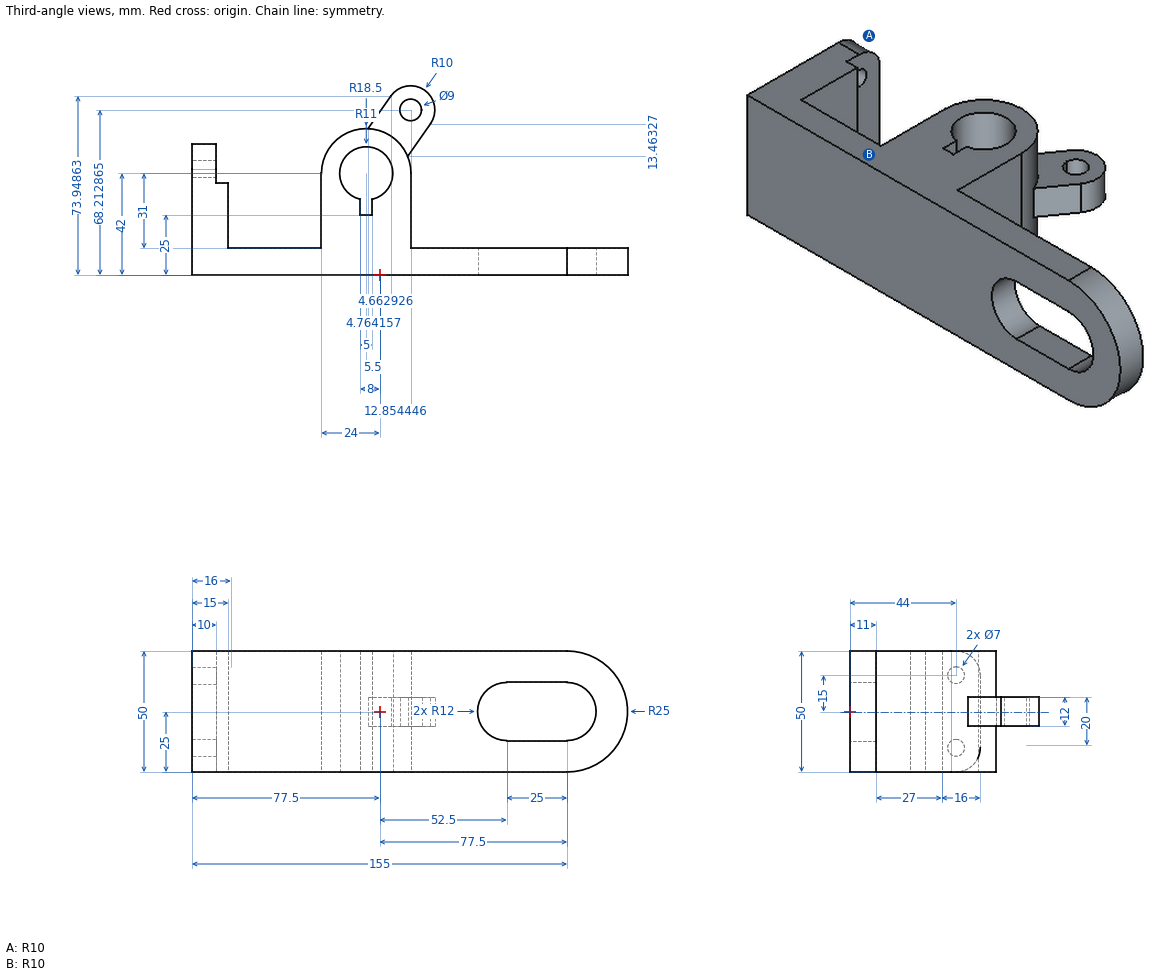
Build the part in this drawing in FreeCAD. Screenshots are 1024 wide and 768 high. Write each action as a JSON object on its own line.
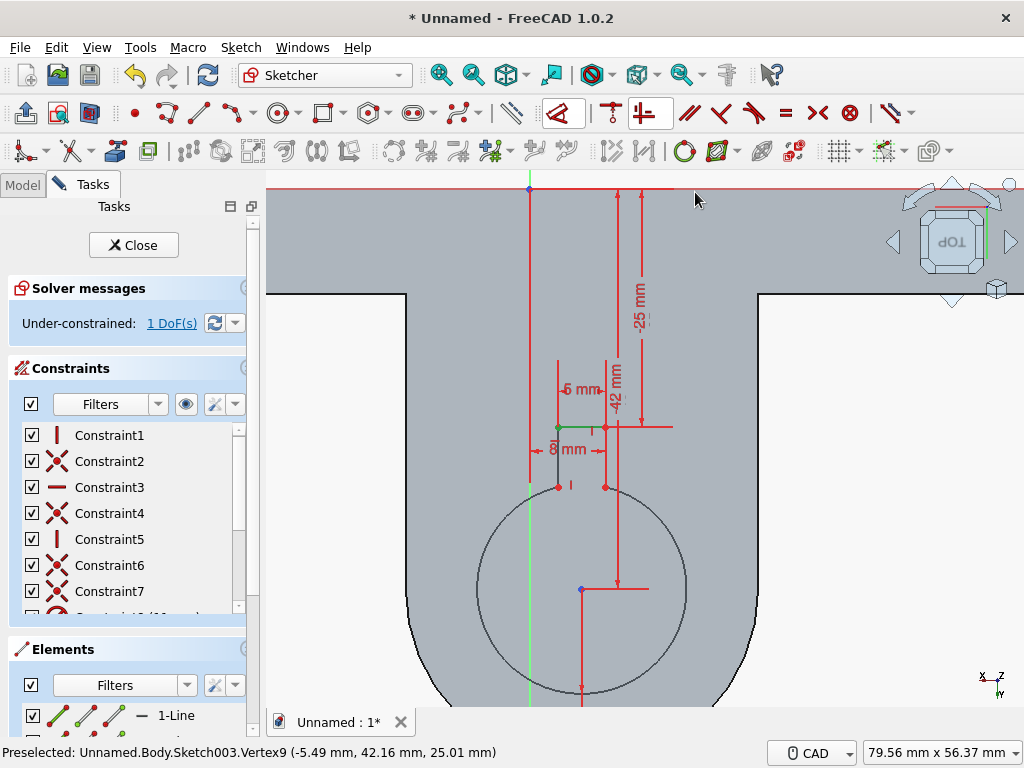
{"action": "left_click", "coordinate": [582, 589]}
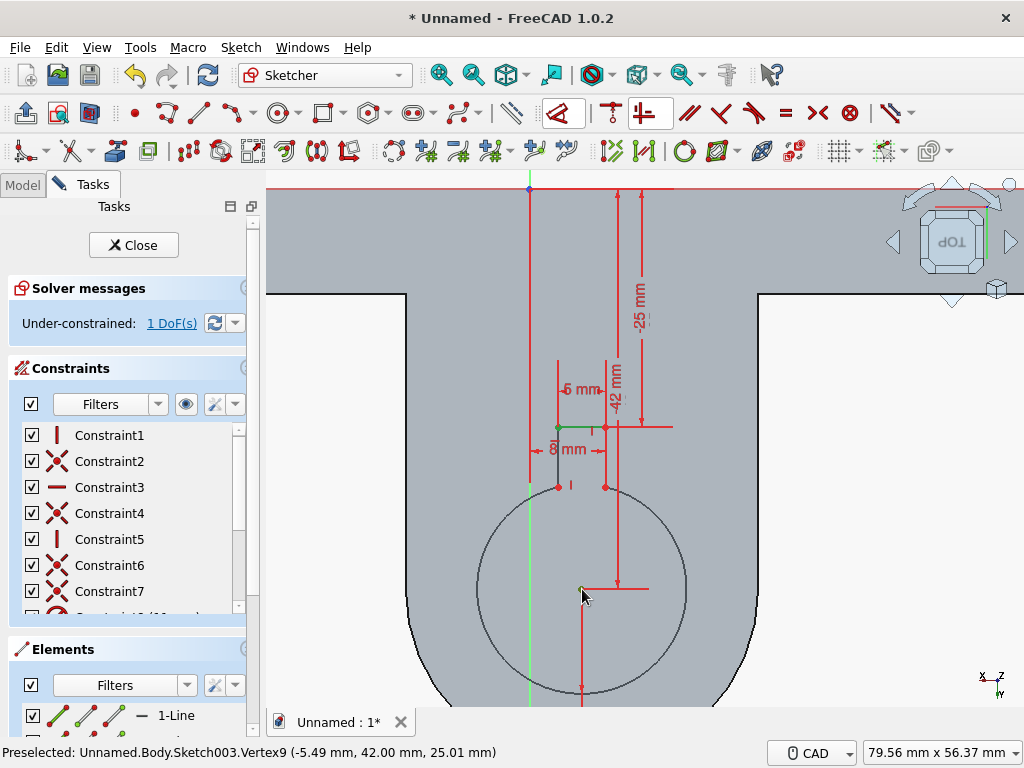
{"action": "left_click", "coordinate": [580, 114]}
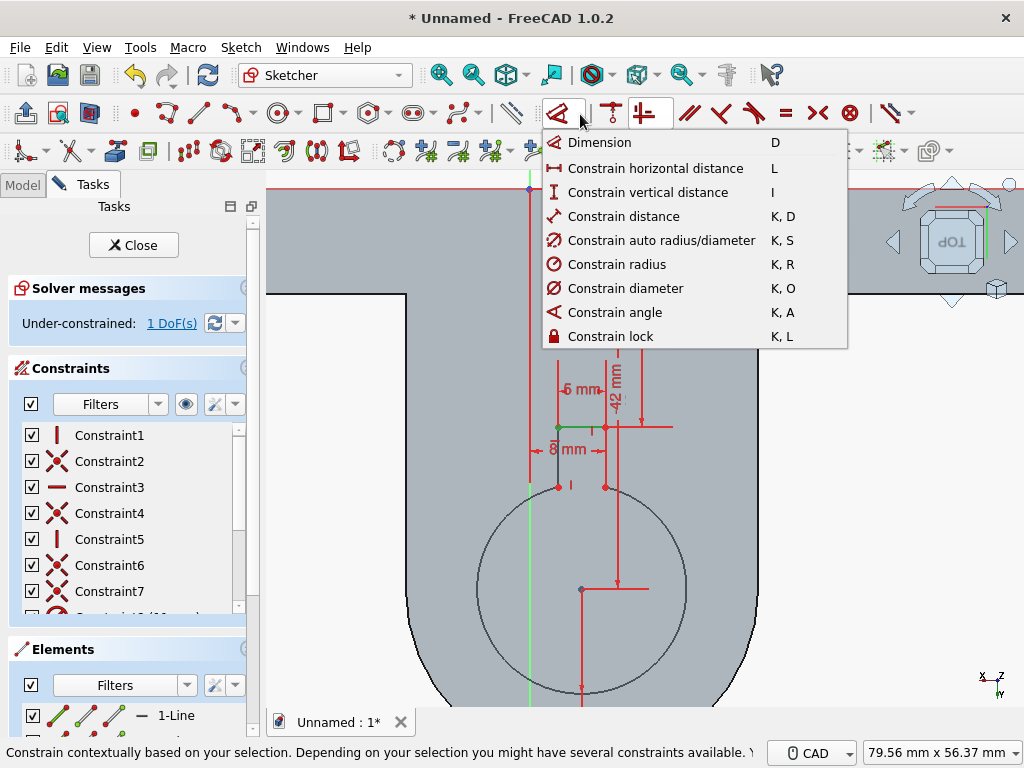
{"action": "left_click", "coordinate": [695, 168]}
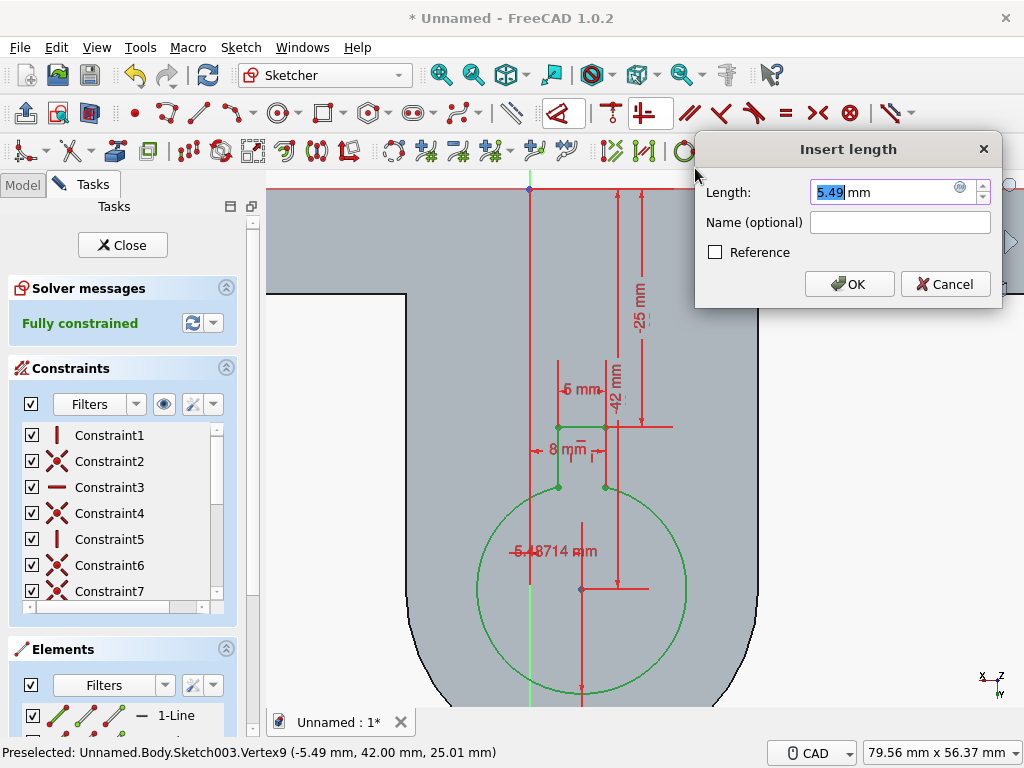
{"action": "type", "text": "5.5"}
{"action": "key", "text": "Return"}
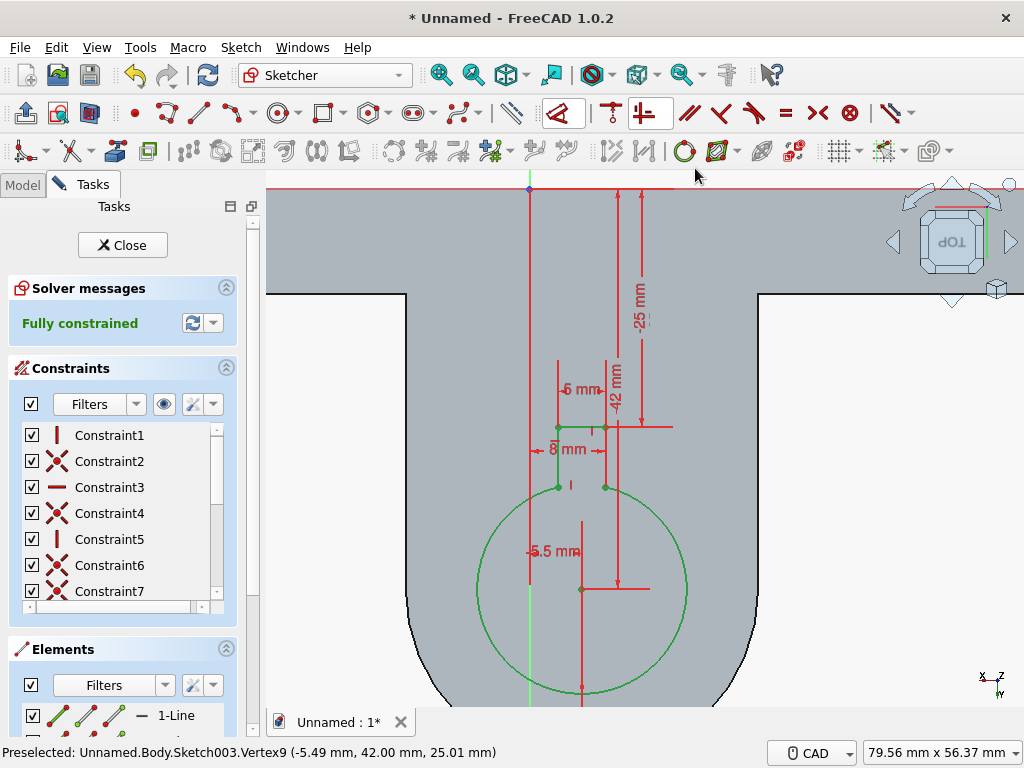
{"action": "left_click", "coordinate": [123, 245]}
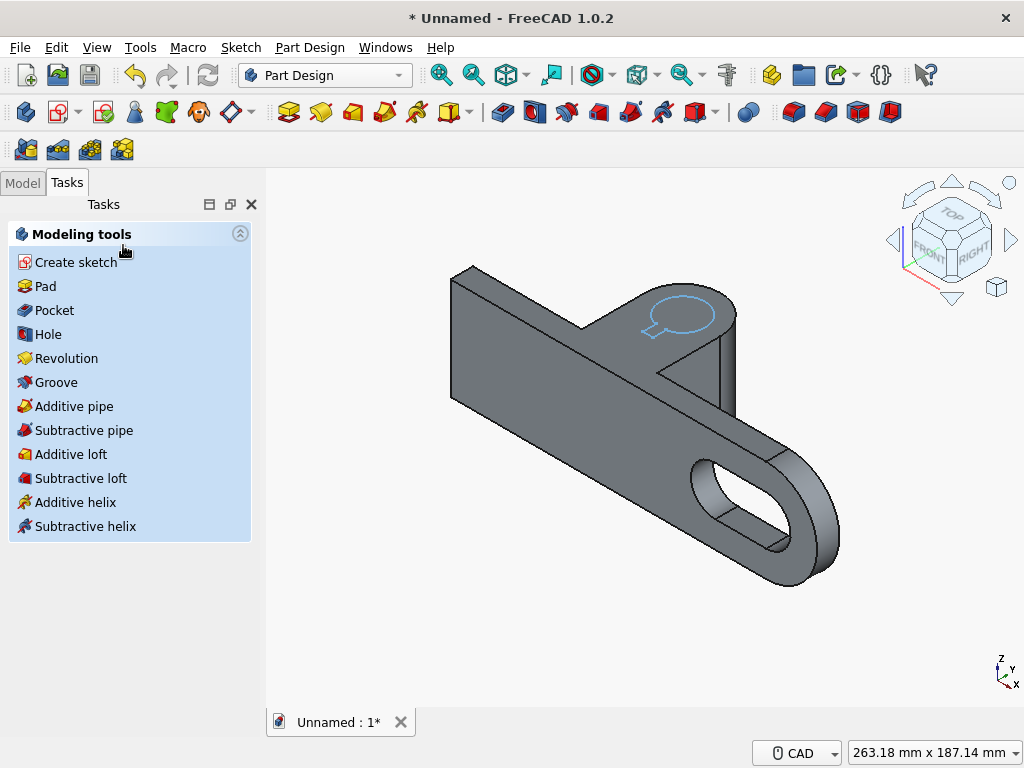
{"action": "left_click", "coordinate": [504, 112]}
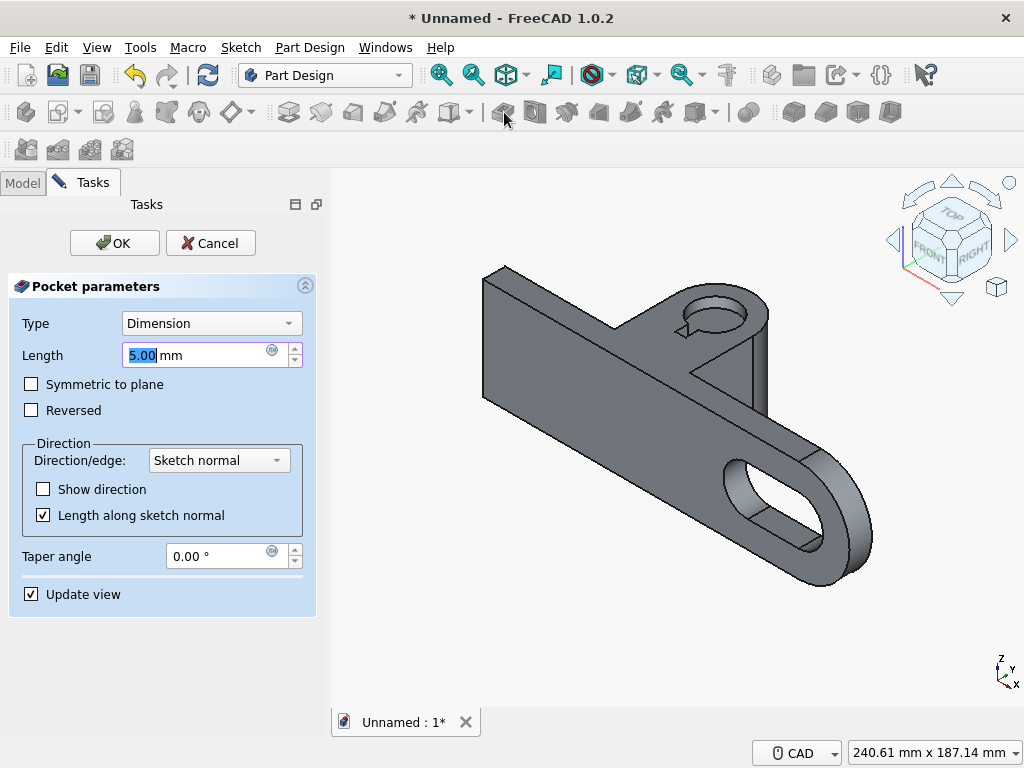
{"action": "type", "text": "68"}
{"action": "key", "text": "Tab"}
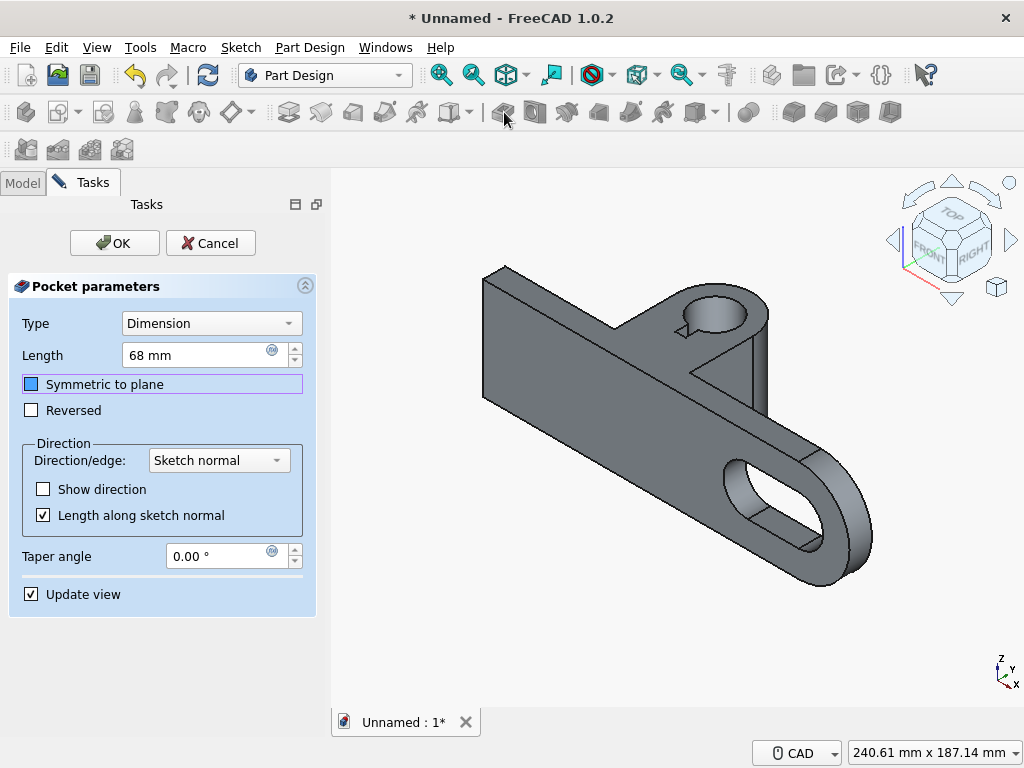
{"action": "left_click", "coordinate": [115, 243]}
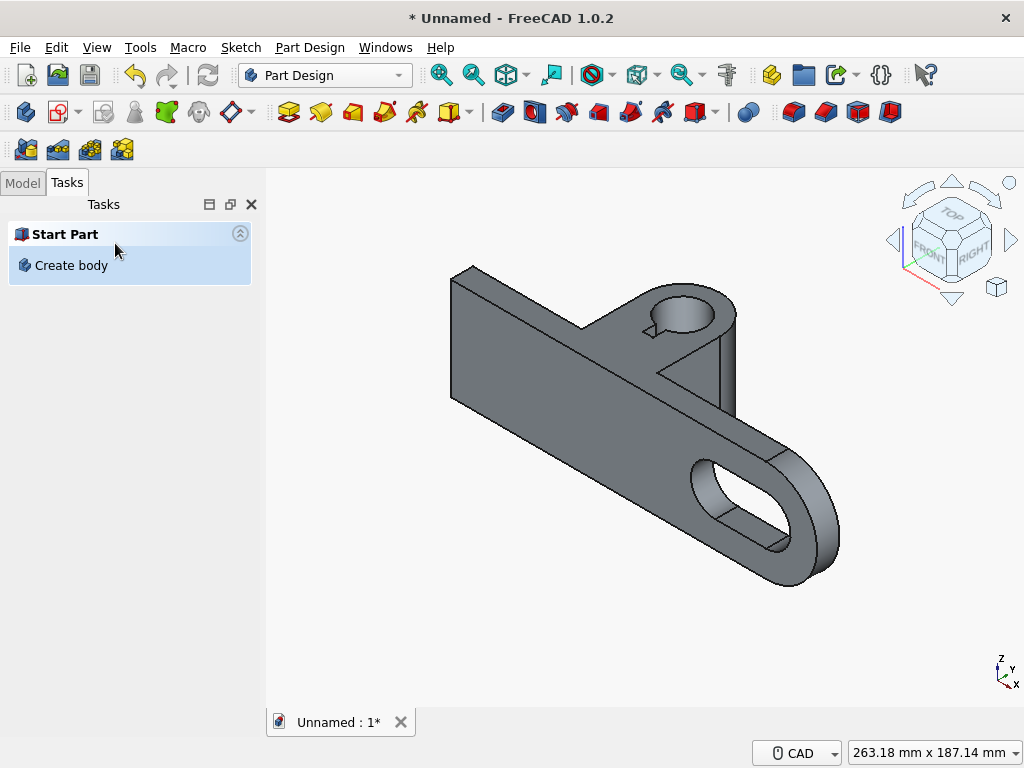
{"action": "left_click", "coordinate": [58, 112]}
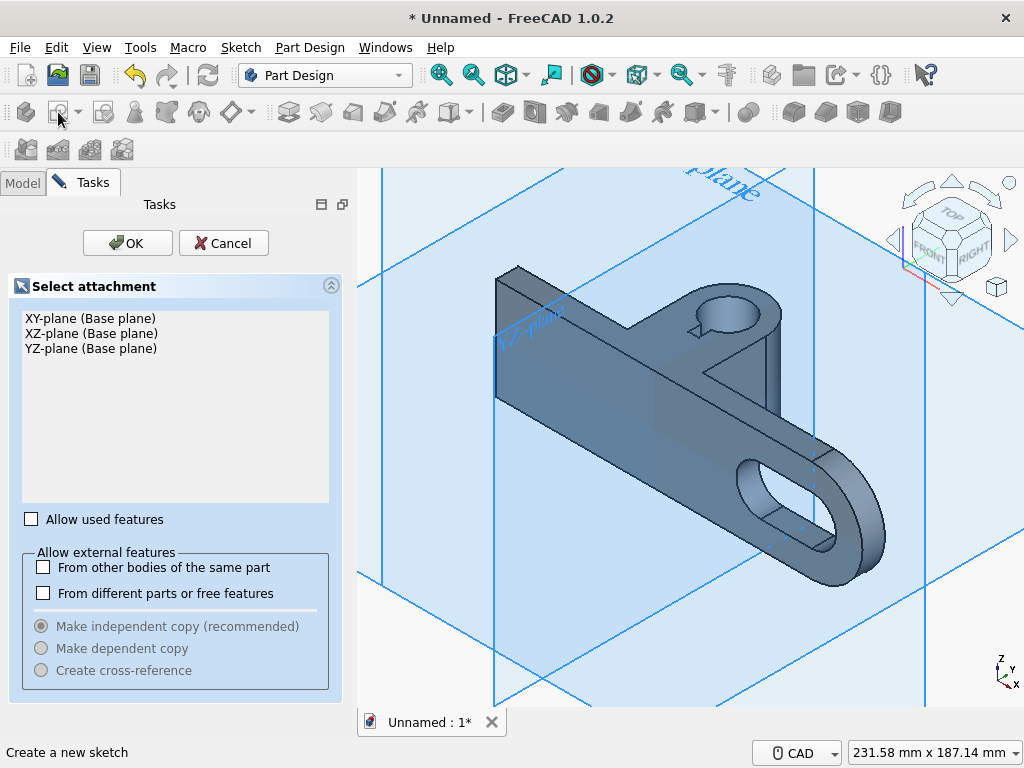
{"action": "left_click", "coordinate": [82, 318]}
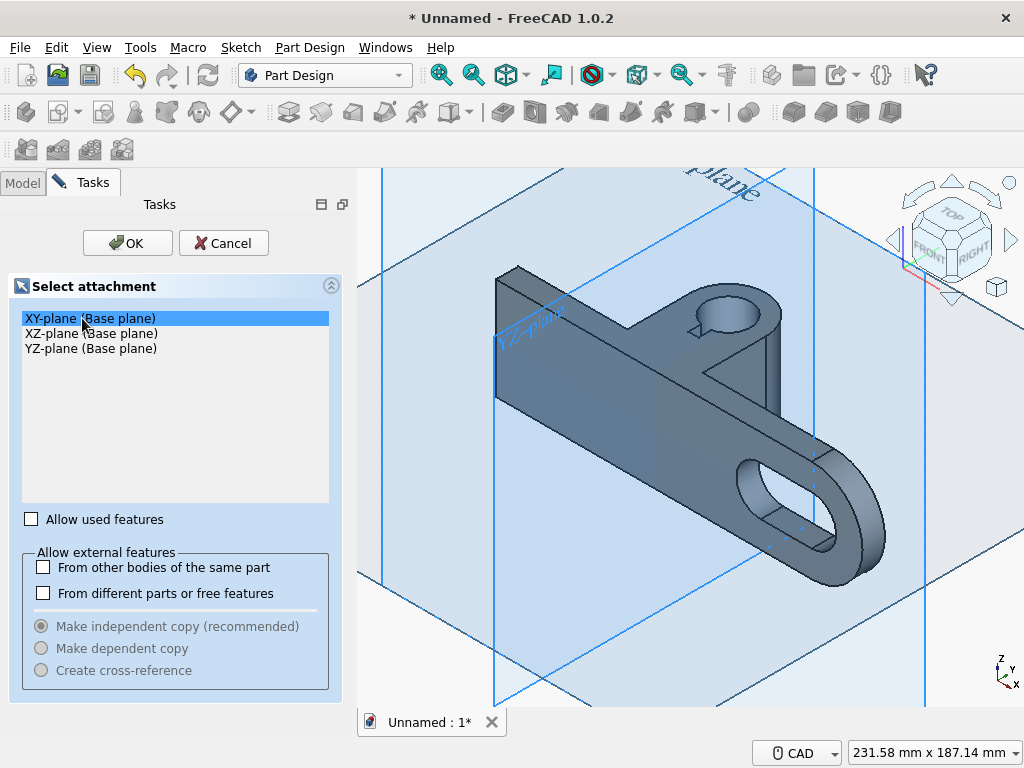
{"action": "left_click", "coordinate": [128, 243]}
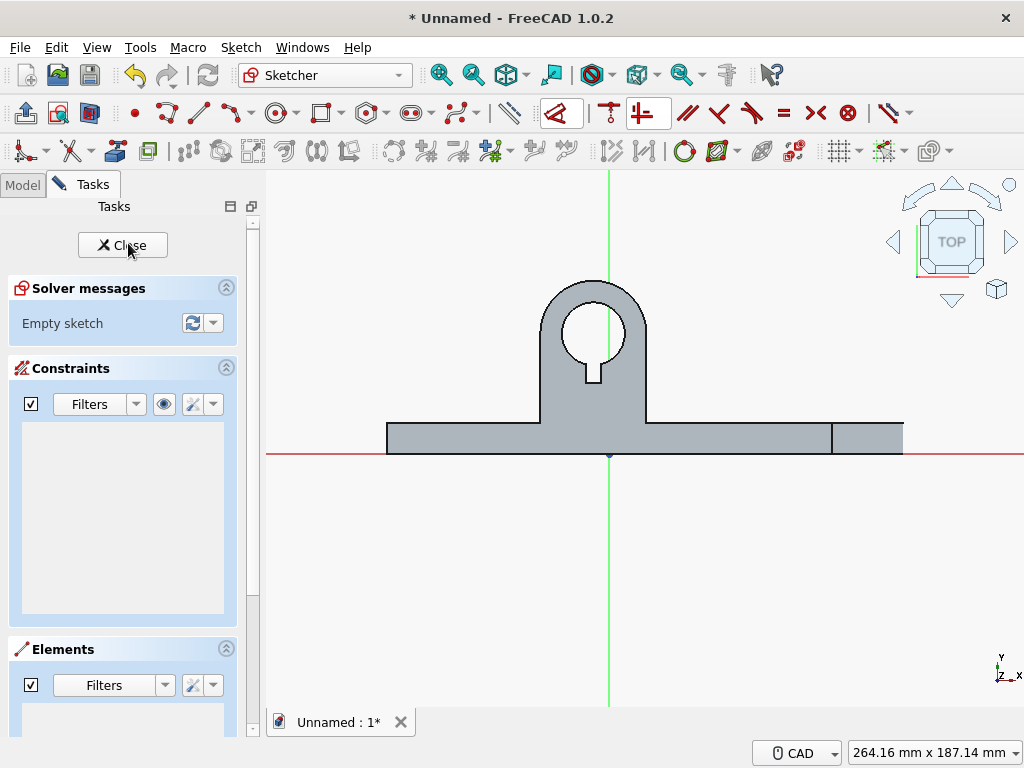
{"action": "key", "text": "q s"}